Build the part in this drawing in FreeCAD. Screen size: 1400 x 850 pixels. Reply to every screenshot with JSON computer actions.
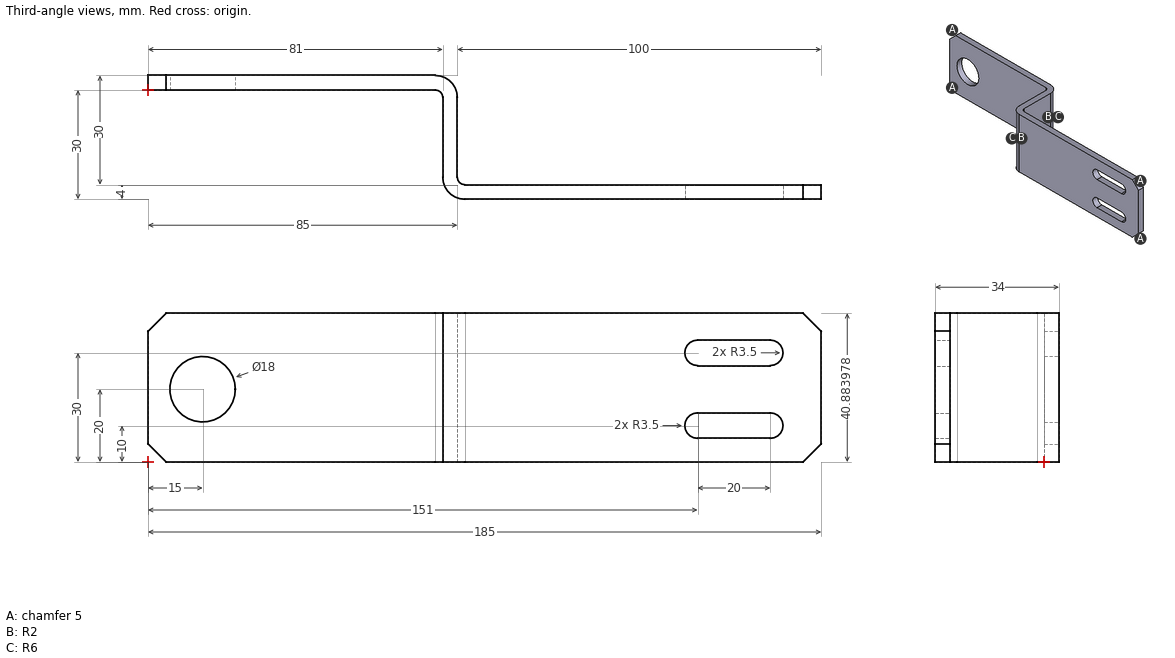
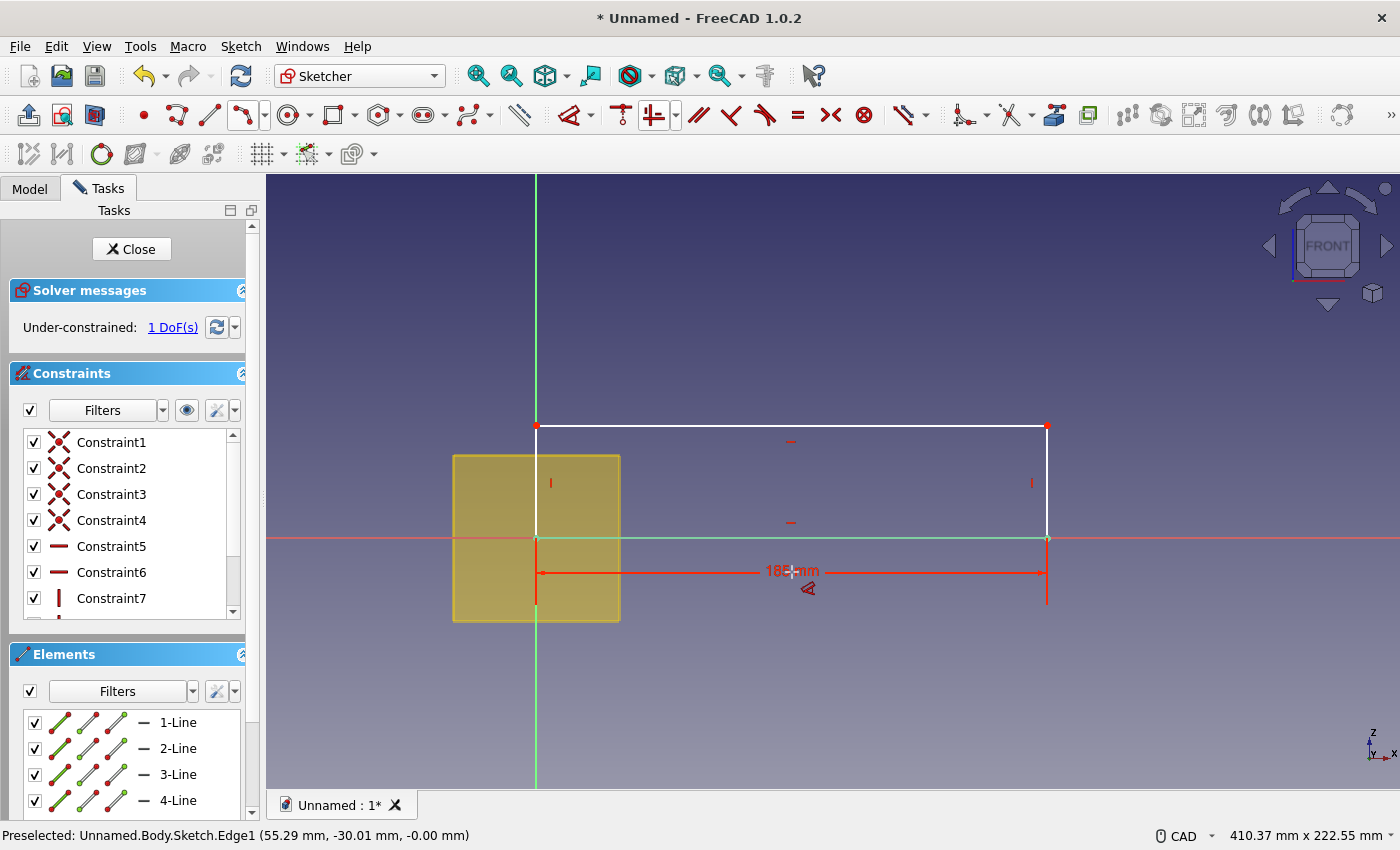
{"action": "left_click", "coordinate": [1047, 505]}
{"action": "left_click", "coordinate": [1081, 482]}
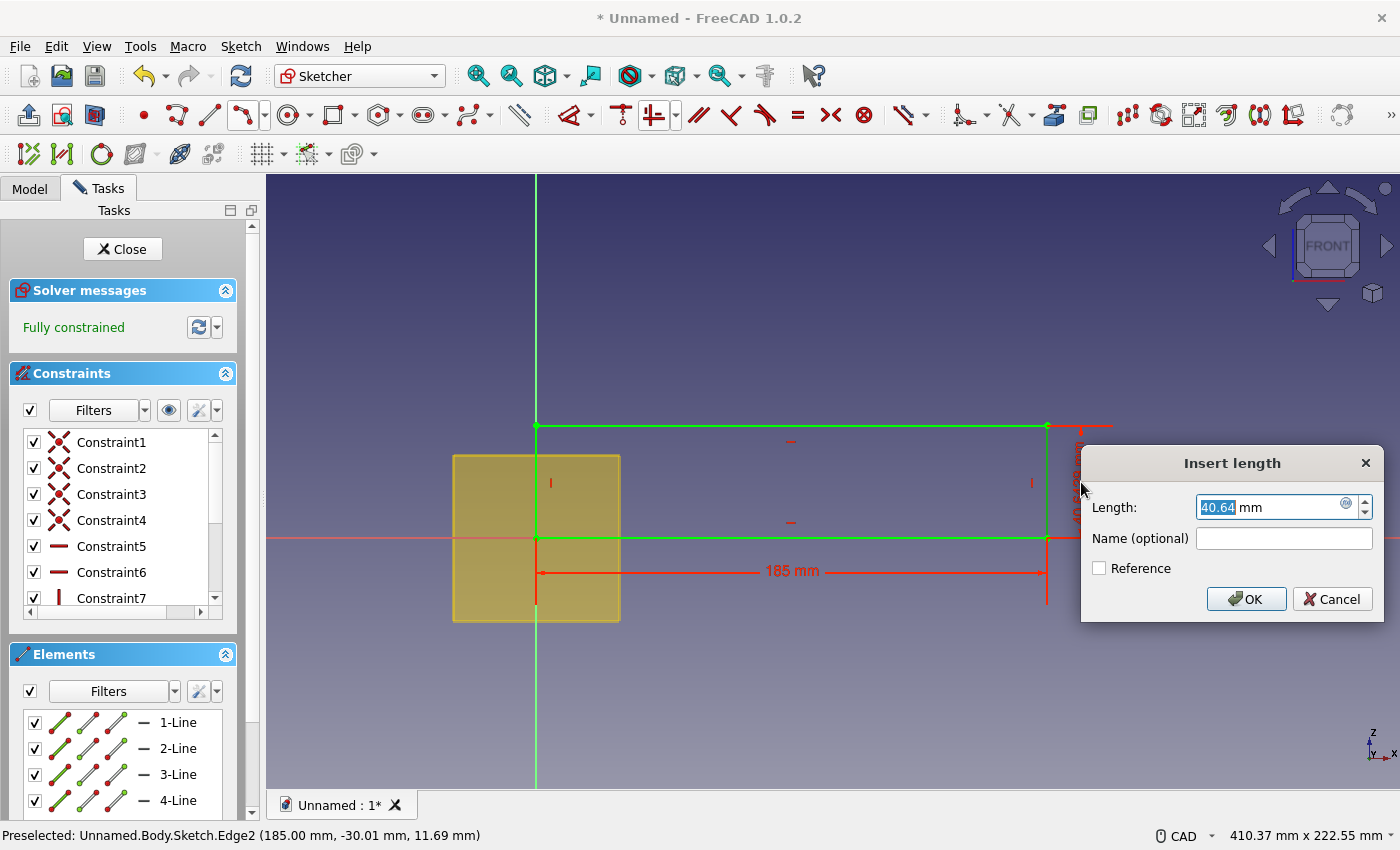
{"action": "type", "text": "40.883978"}
{"action": "key", "text": "Return"}
{"action": "key", "text": "Escape"}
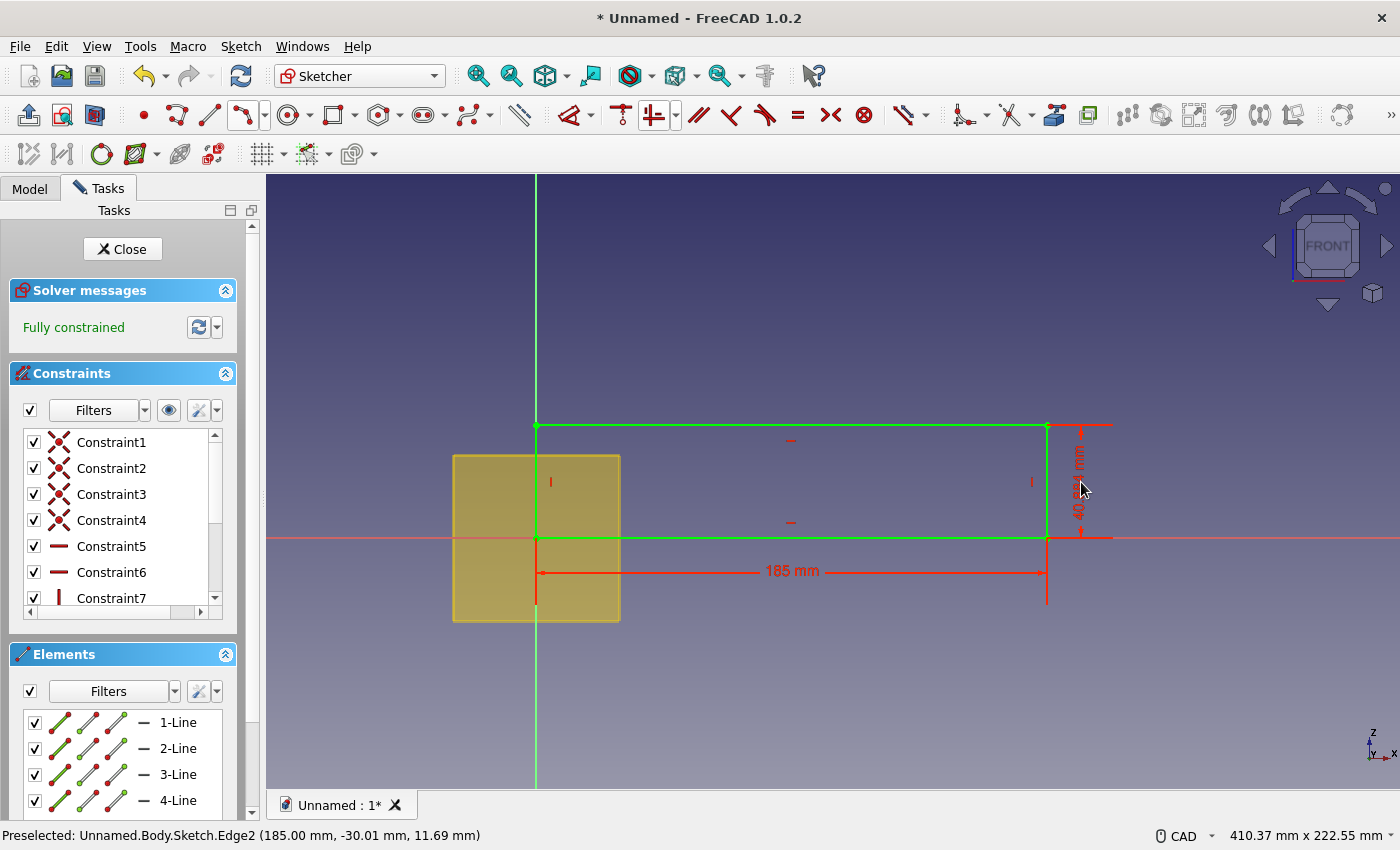
{"action": "left_click", "coordinate": [123, 249]}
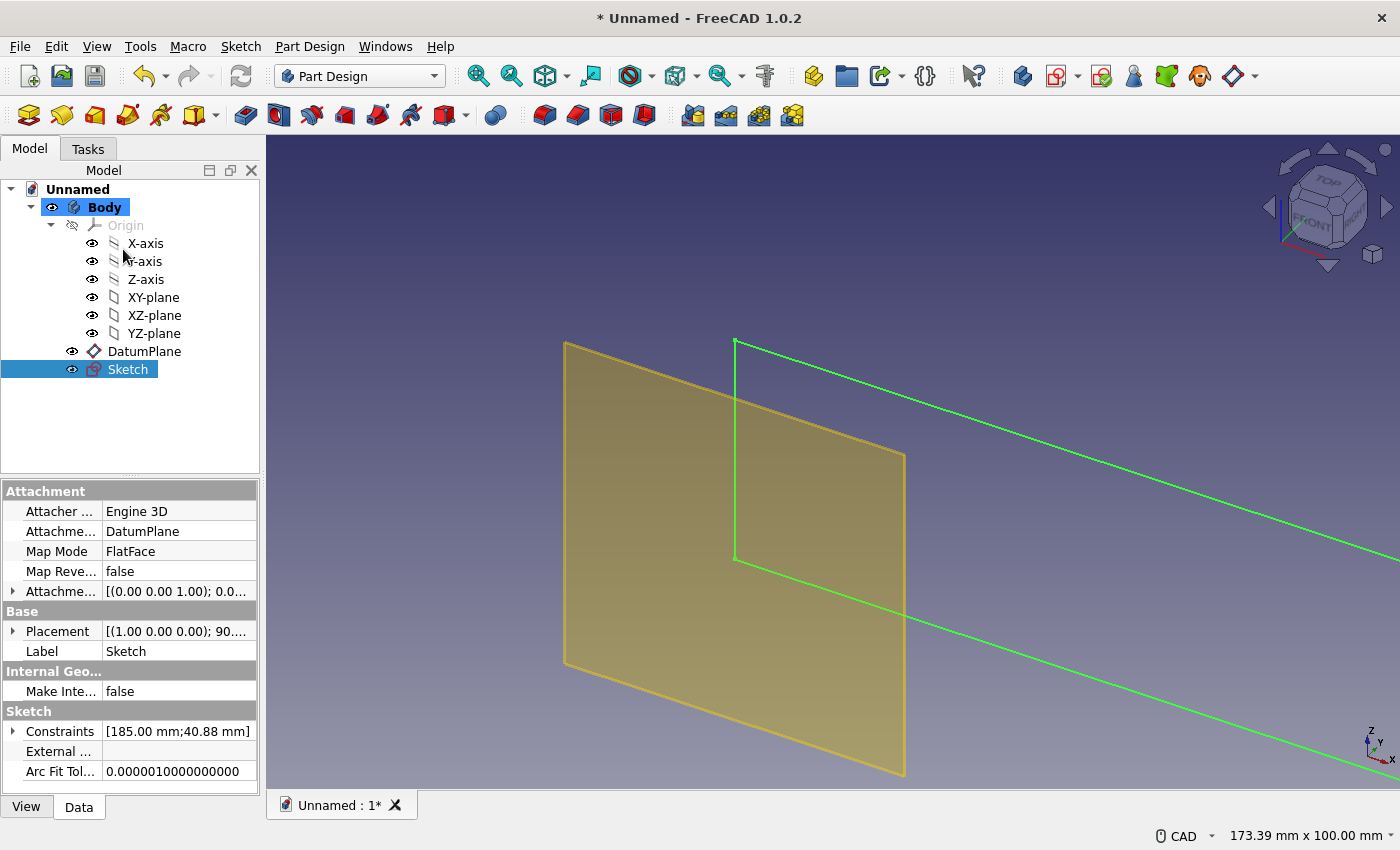
{"action": "left_click", "coordinate": [29, 116]}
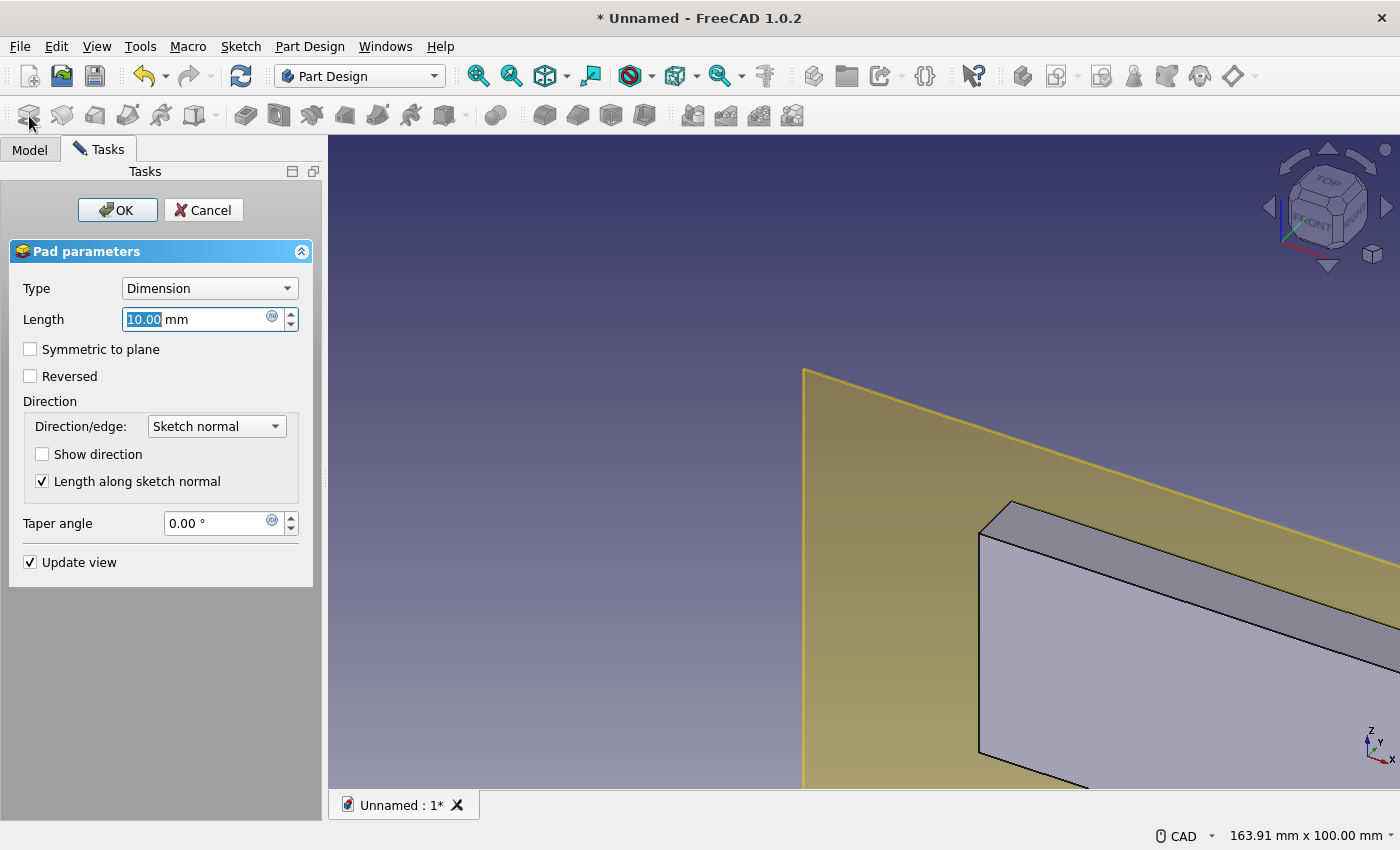
{"action": "type", "text": "34"}
{"action": "key", "text": "Tab"}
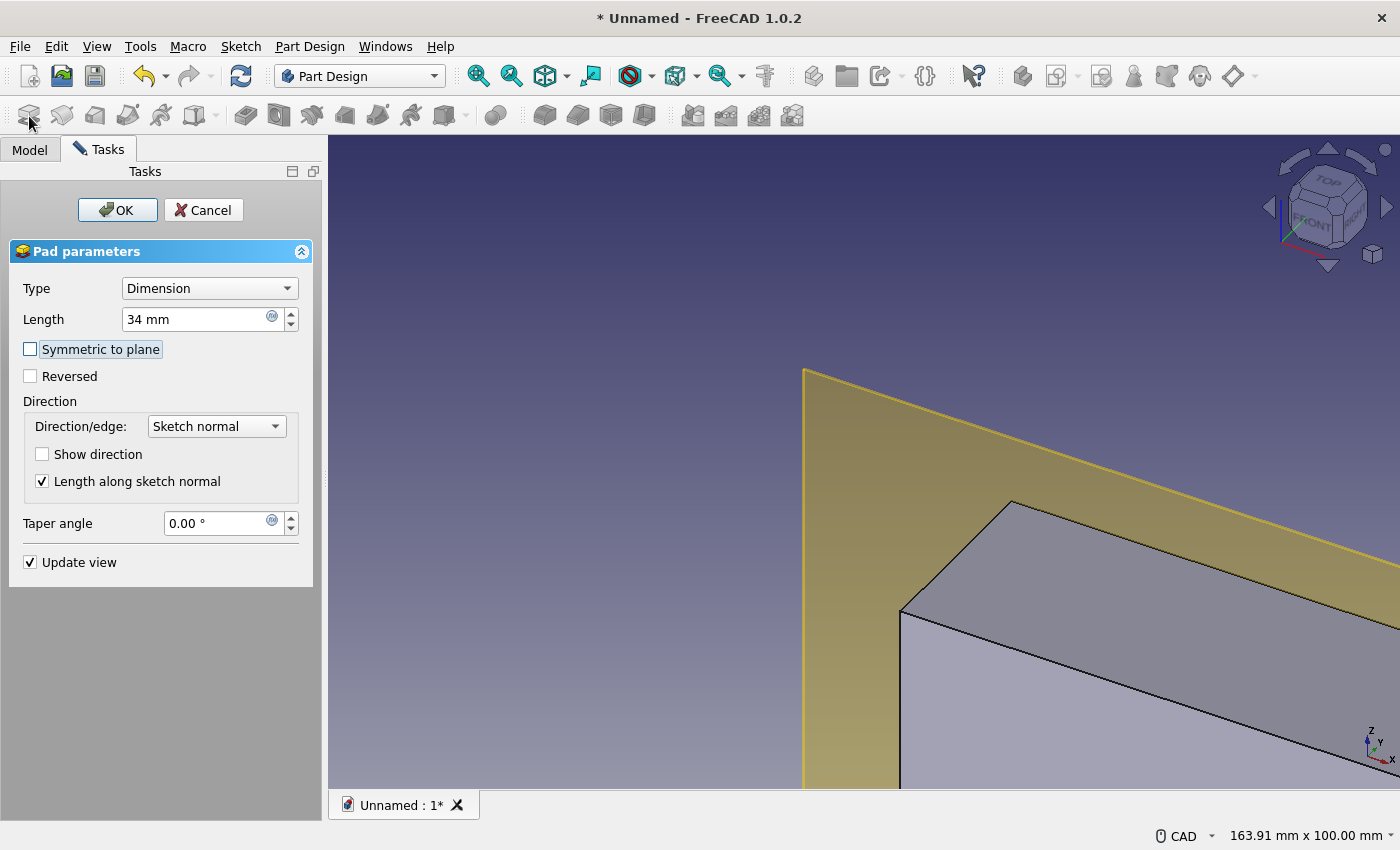
{"action": "left_click", "coordinate": [31, 376]}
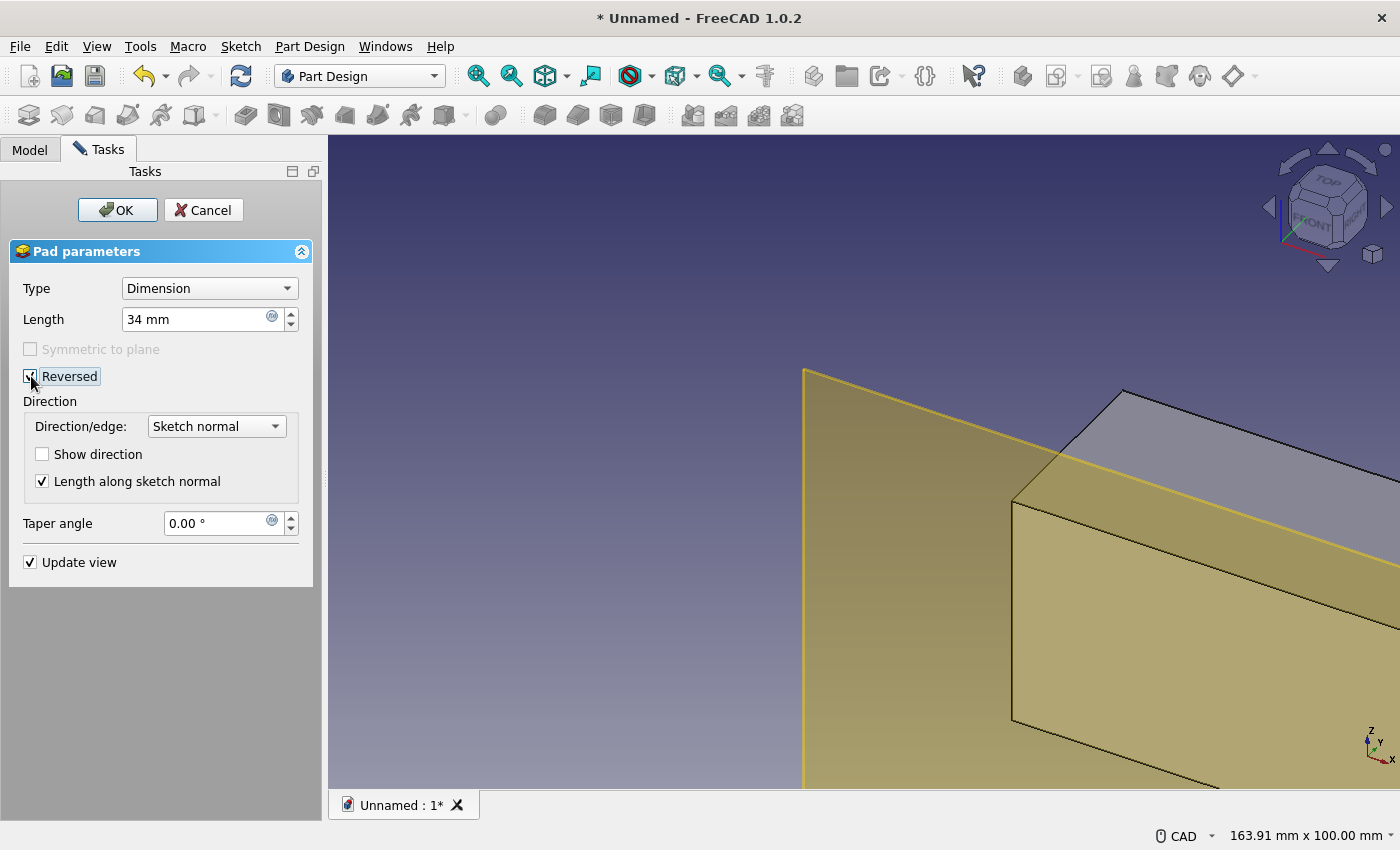
{"action": "left_click", "coordinate": [118, 210]}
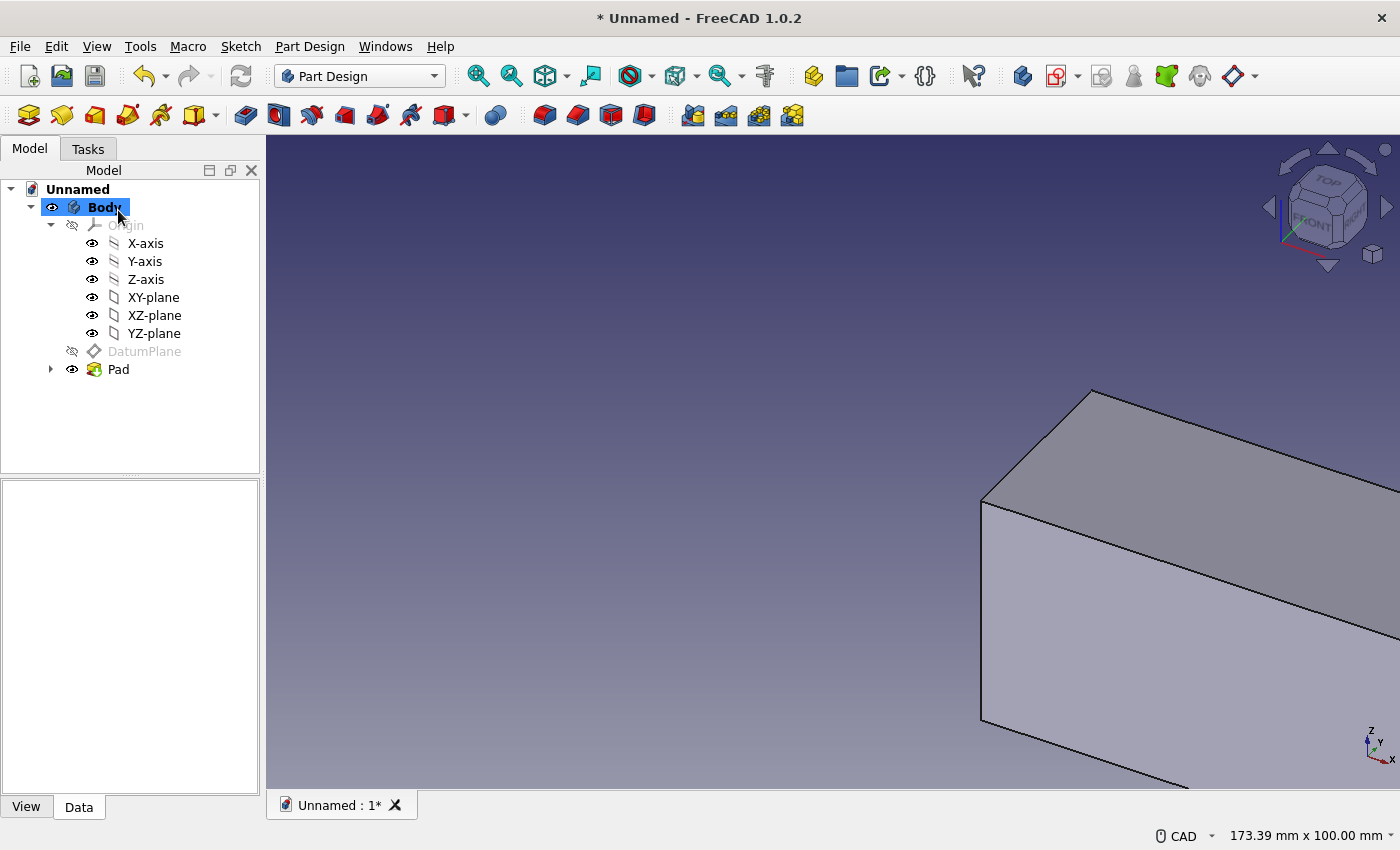
{"action": "left_click", "coordinate": [479, 76]}